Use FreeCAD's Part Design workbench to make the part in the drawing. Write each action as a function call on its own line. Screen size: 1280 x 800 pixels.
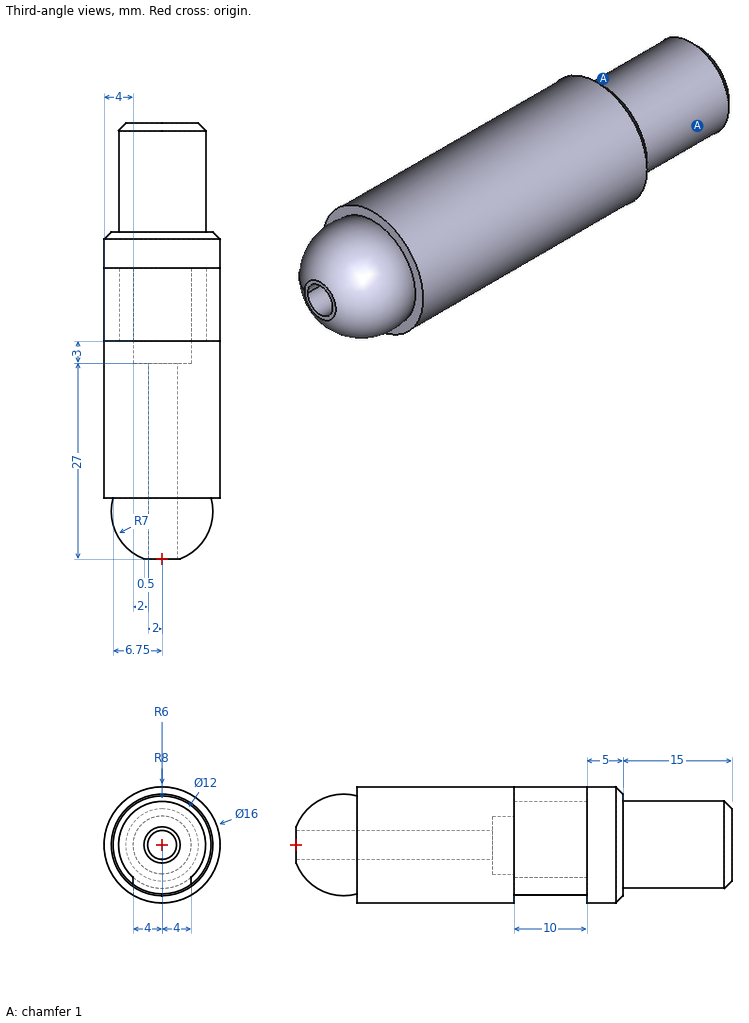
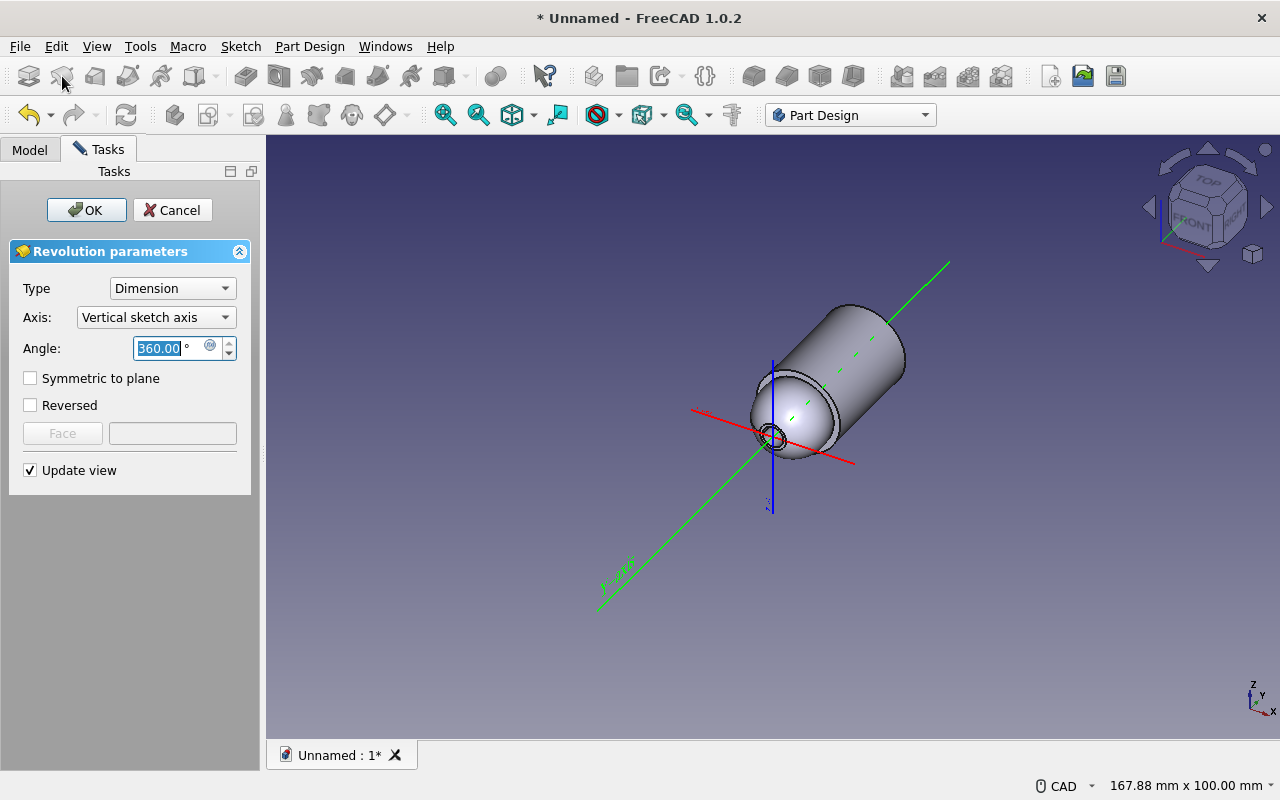
click(87, 210)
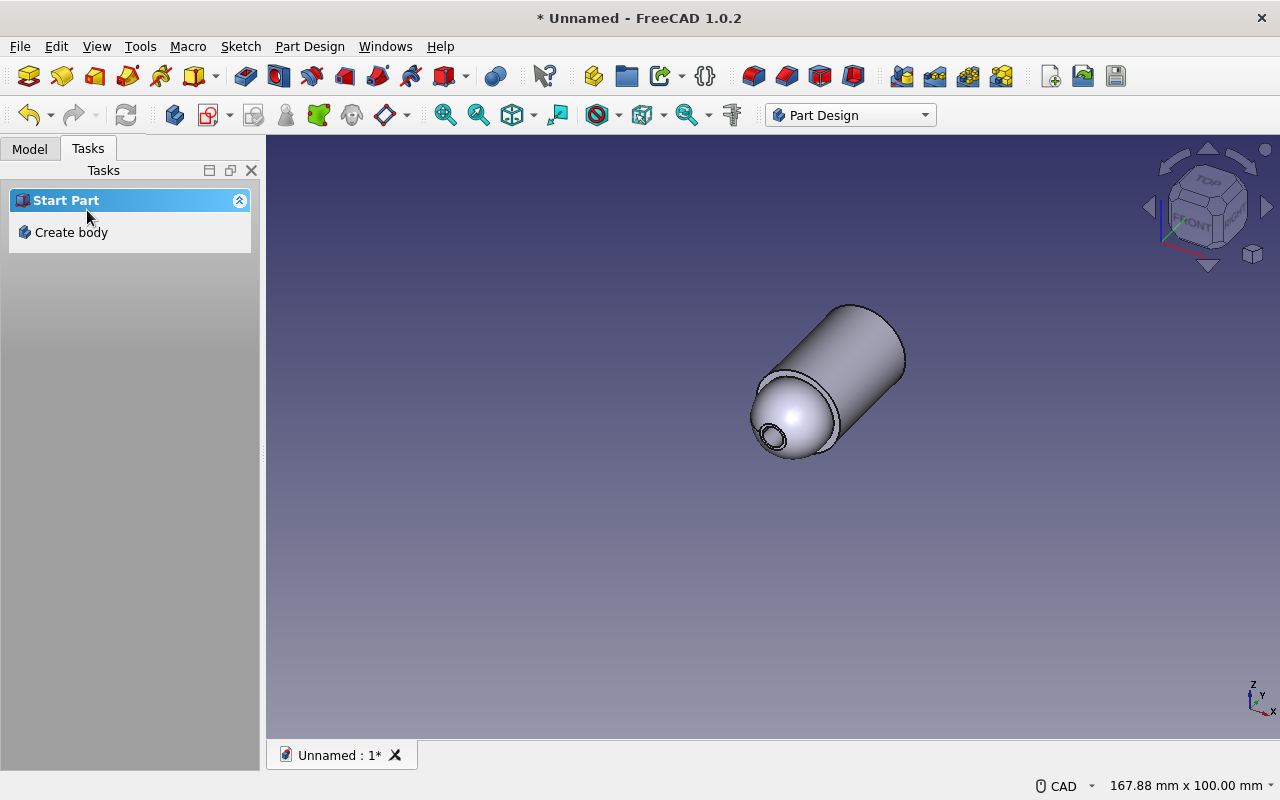
click(446, 116)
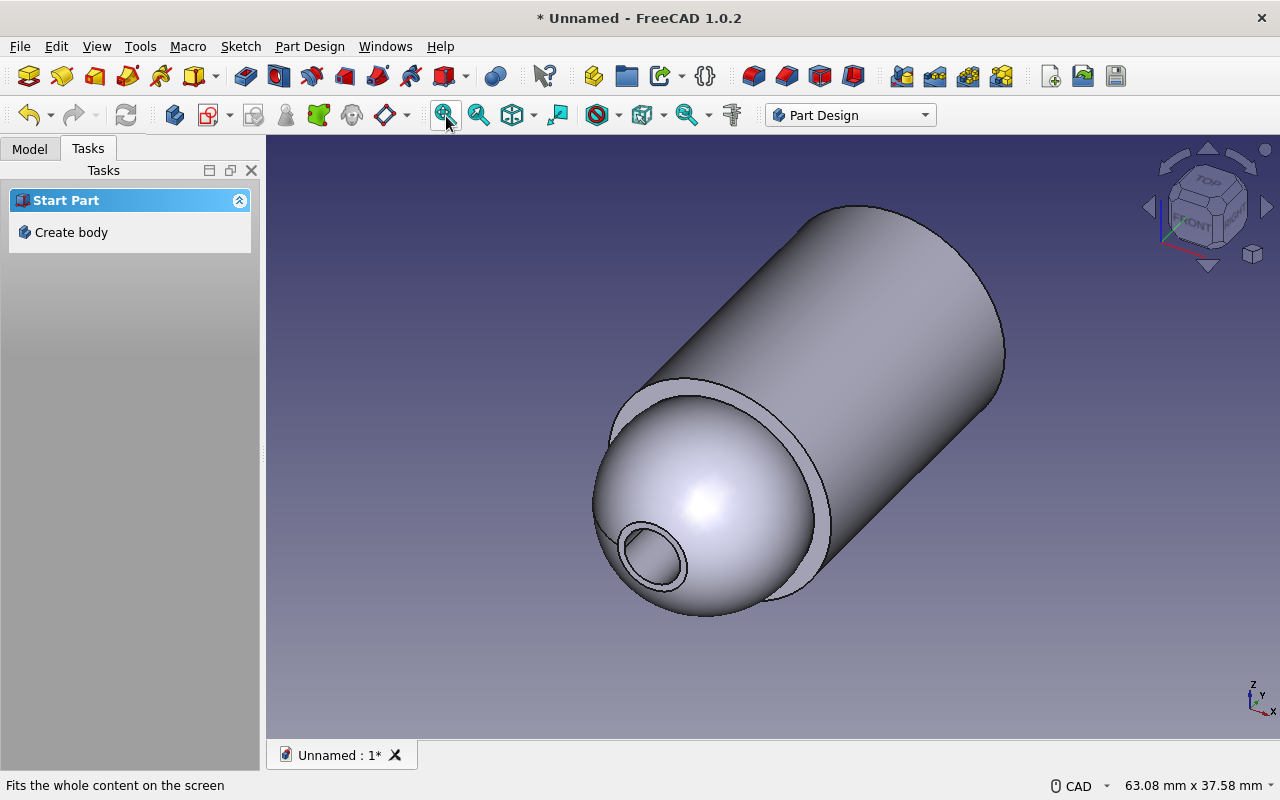
key(4)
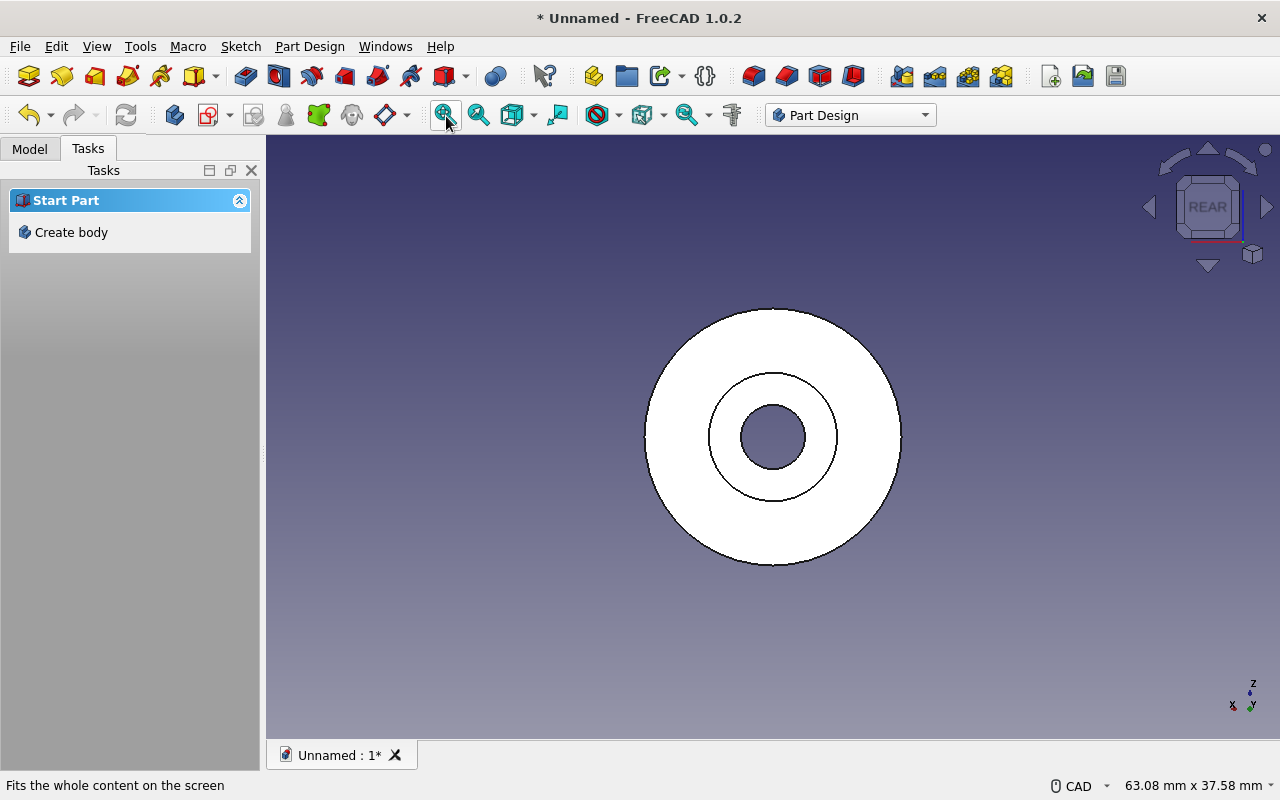
click(446, 116)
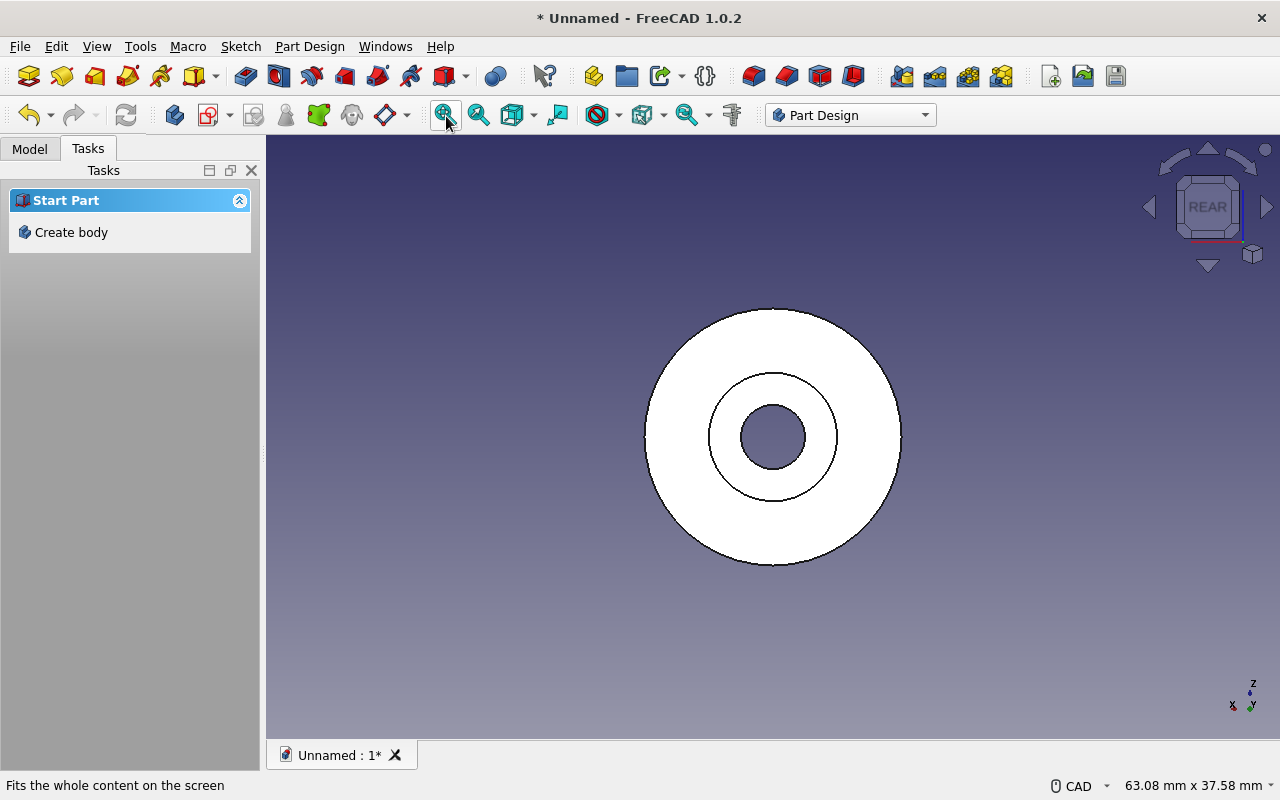
click(700, 509)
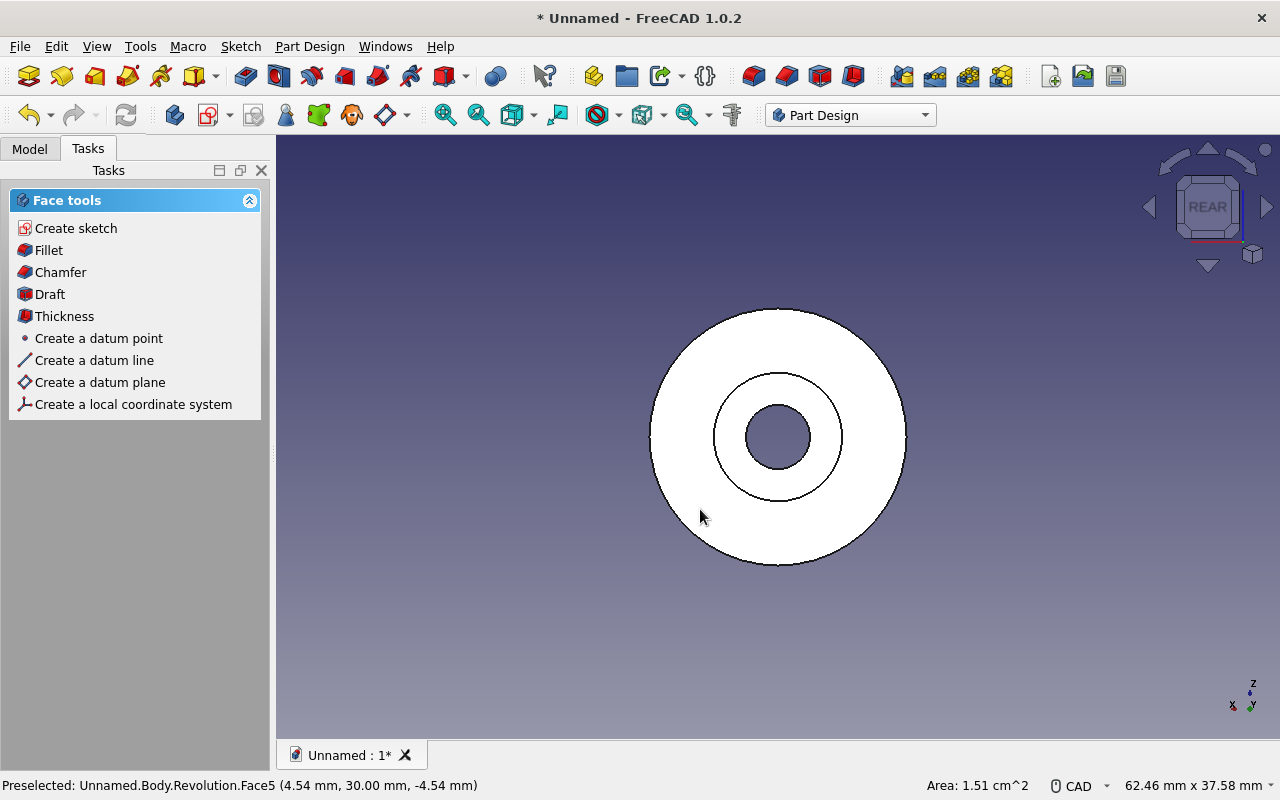
click(208, 116)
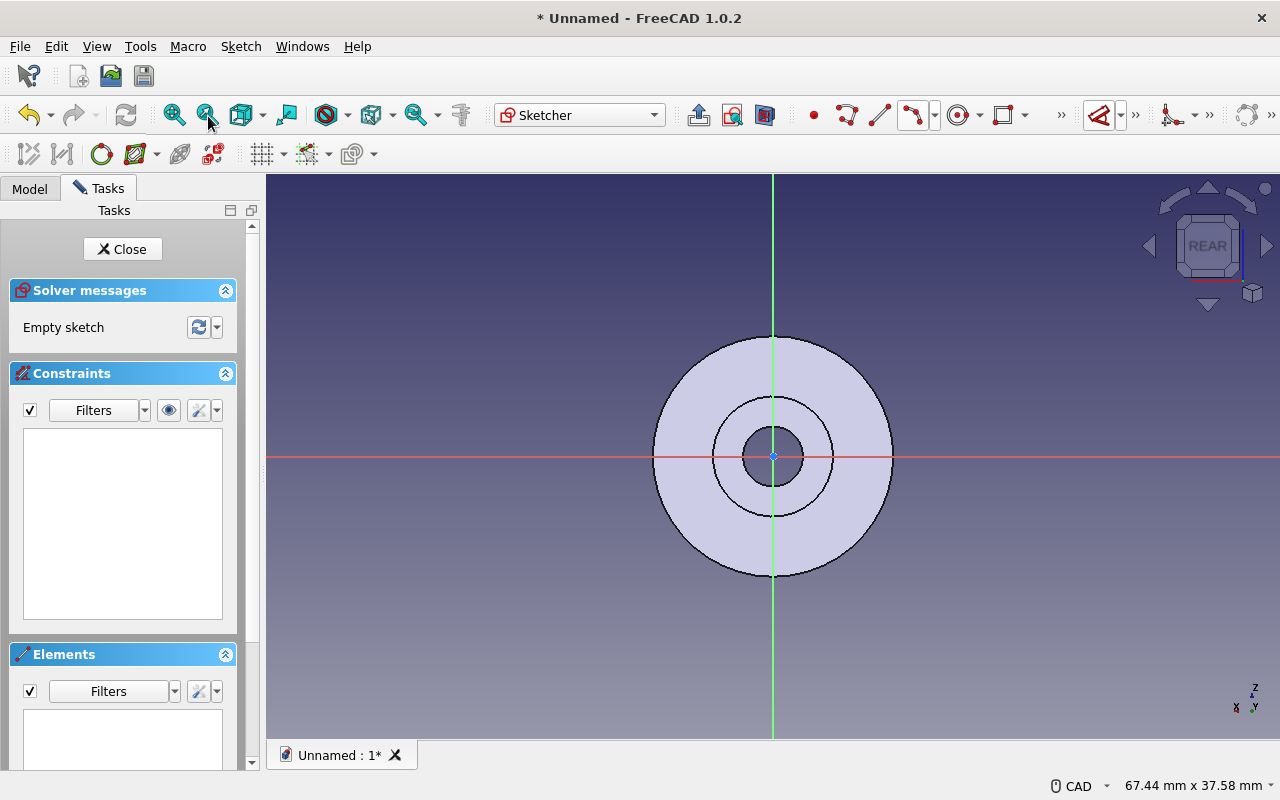
scroll(912, 432, up, 2)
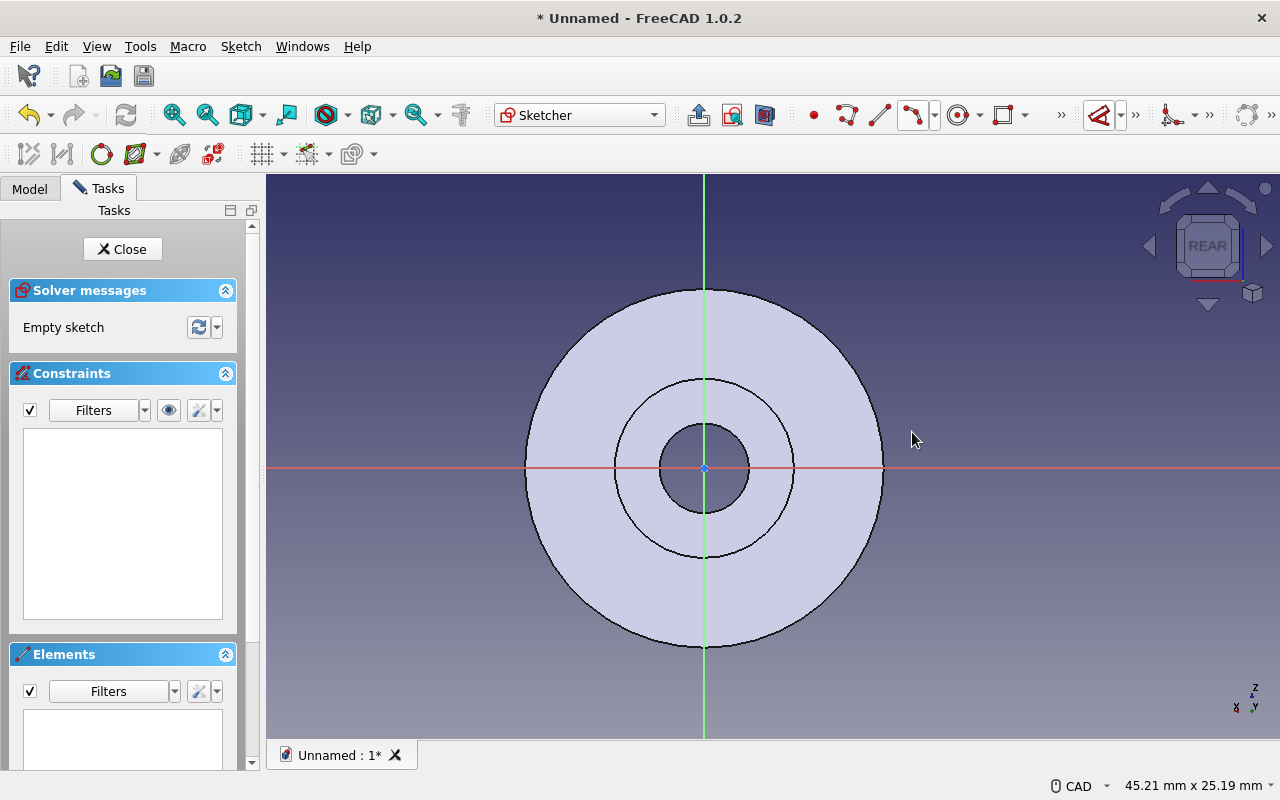
click(880, 116)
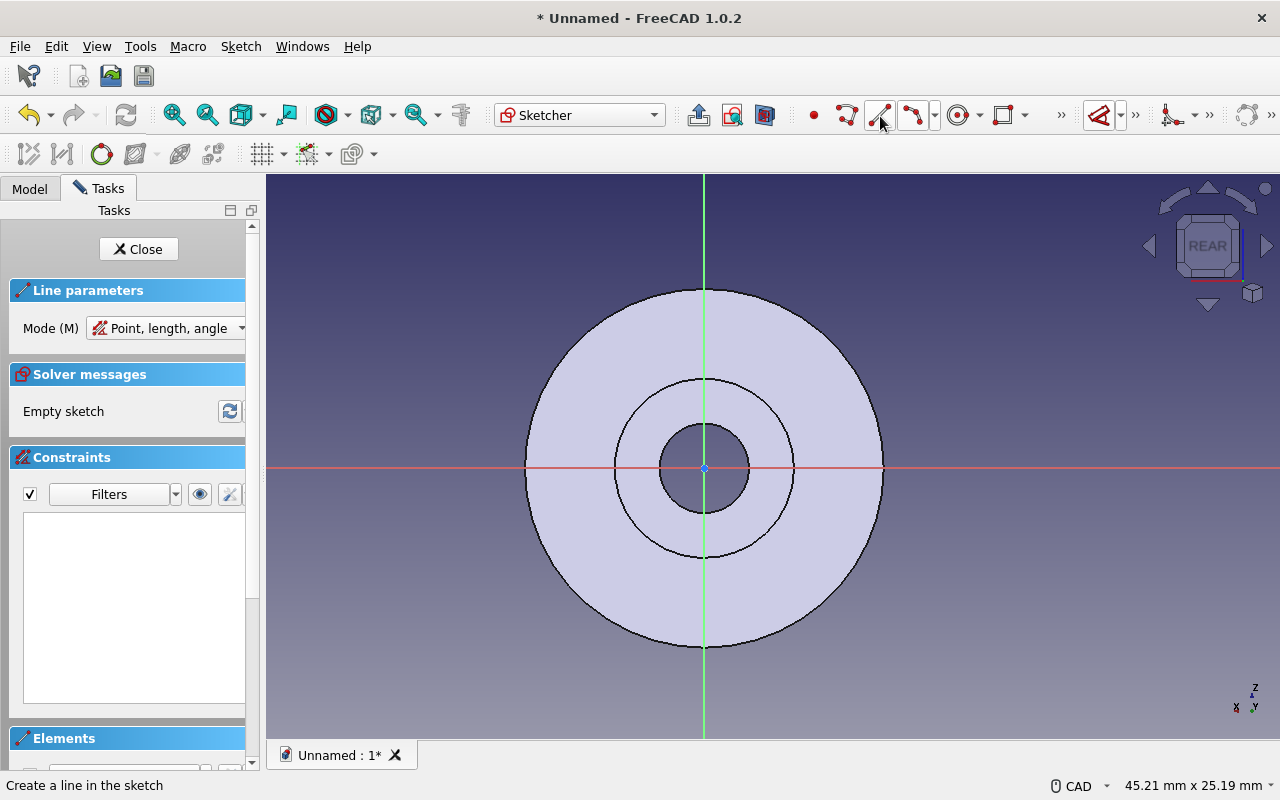
click(794, 569)
click(794, 624)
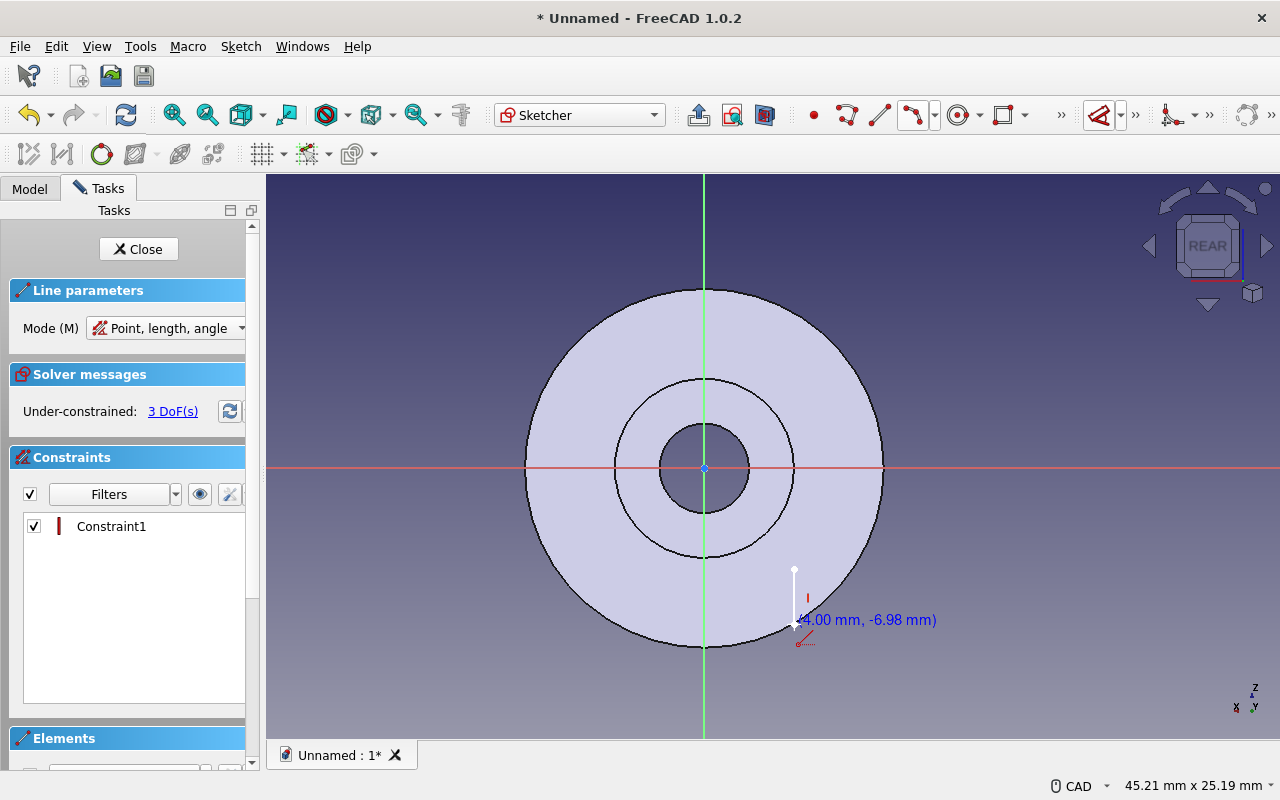
click(615, 624)
click(615, 569)